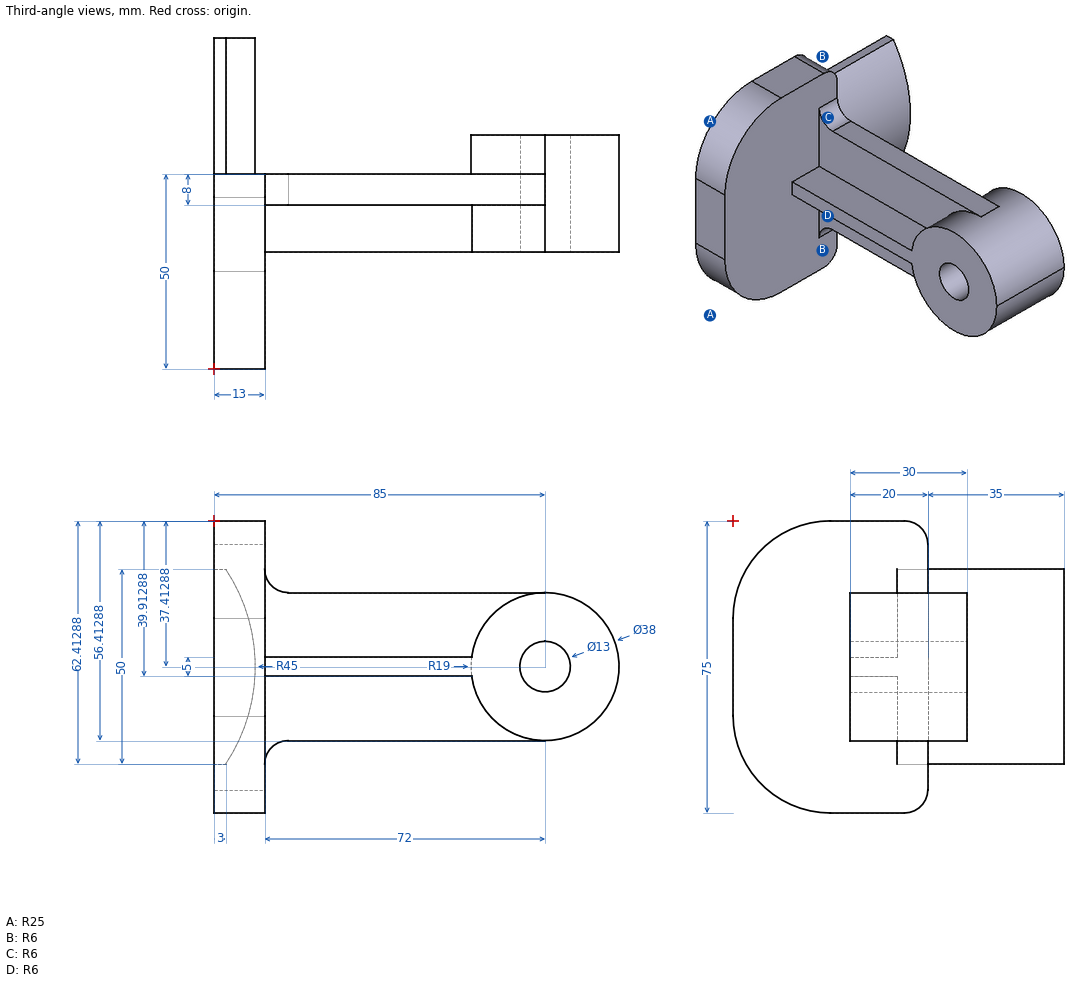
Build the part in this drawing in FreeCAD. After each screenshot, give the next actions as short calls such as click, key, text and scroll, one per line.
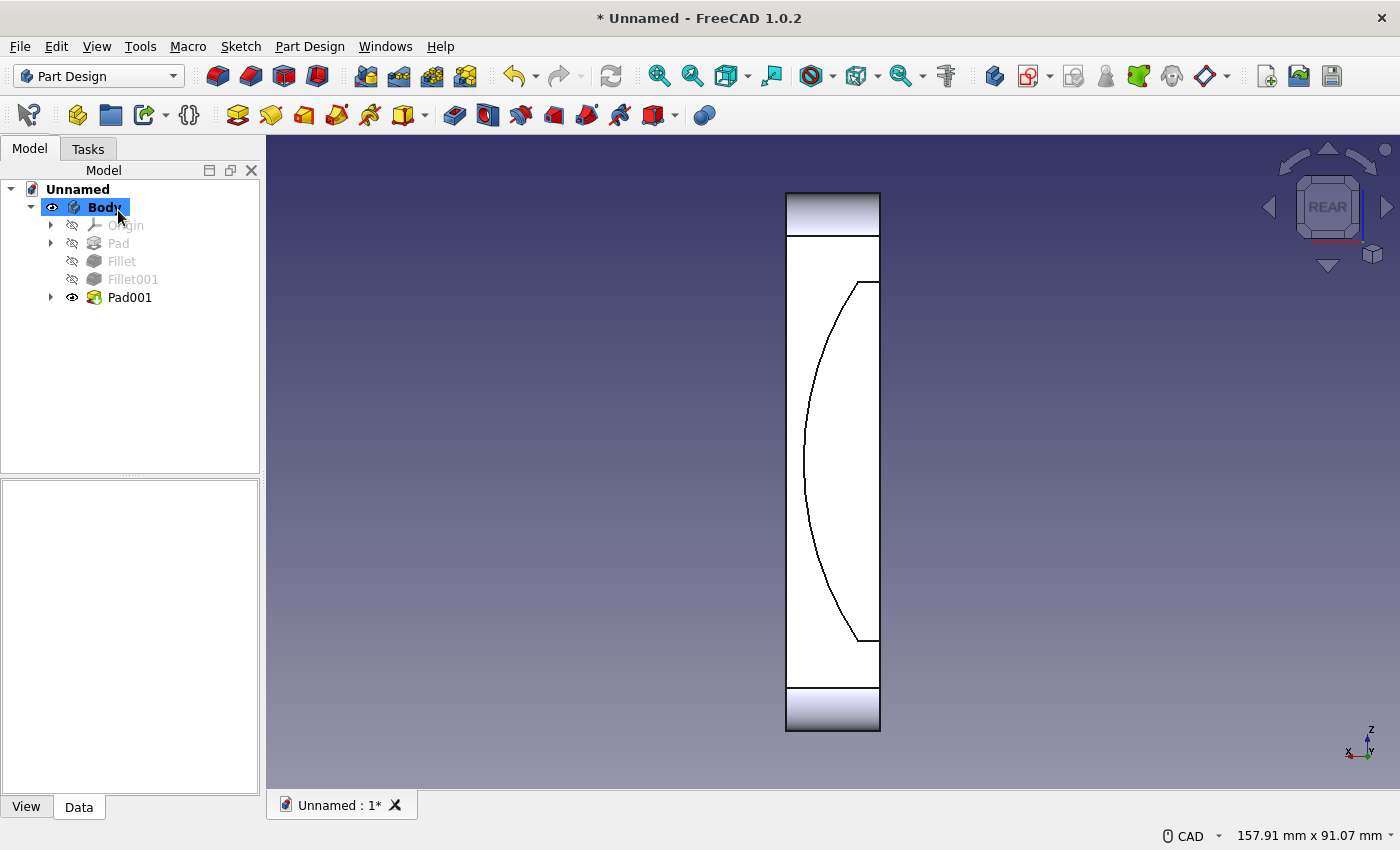
click(995, 76)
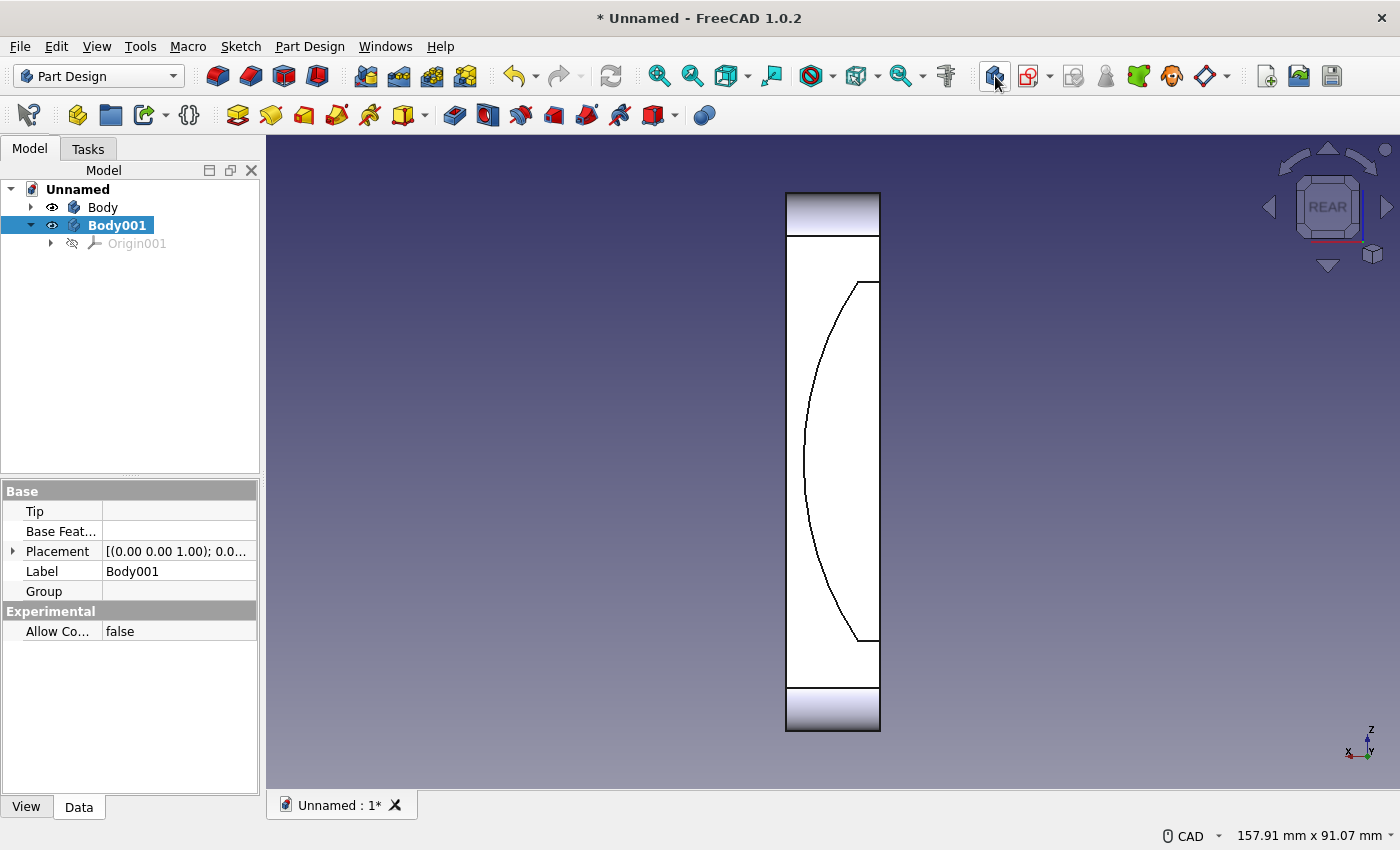
click(51, 243)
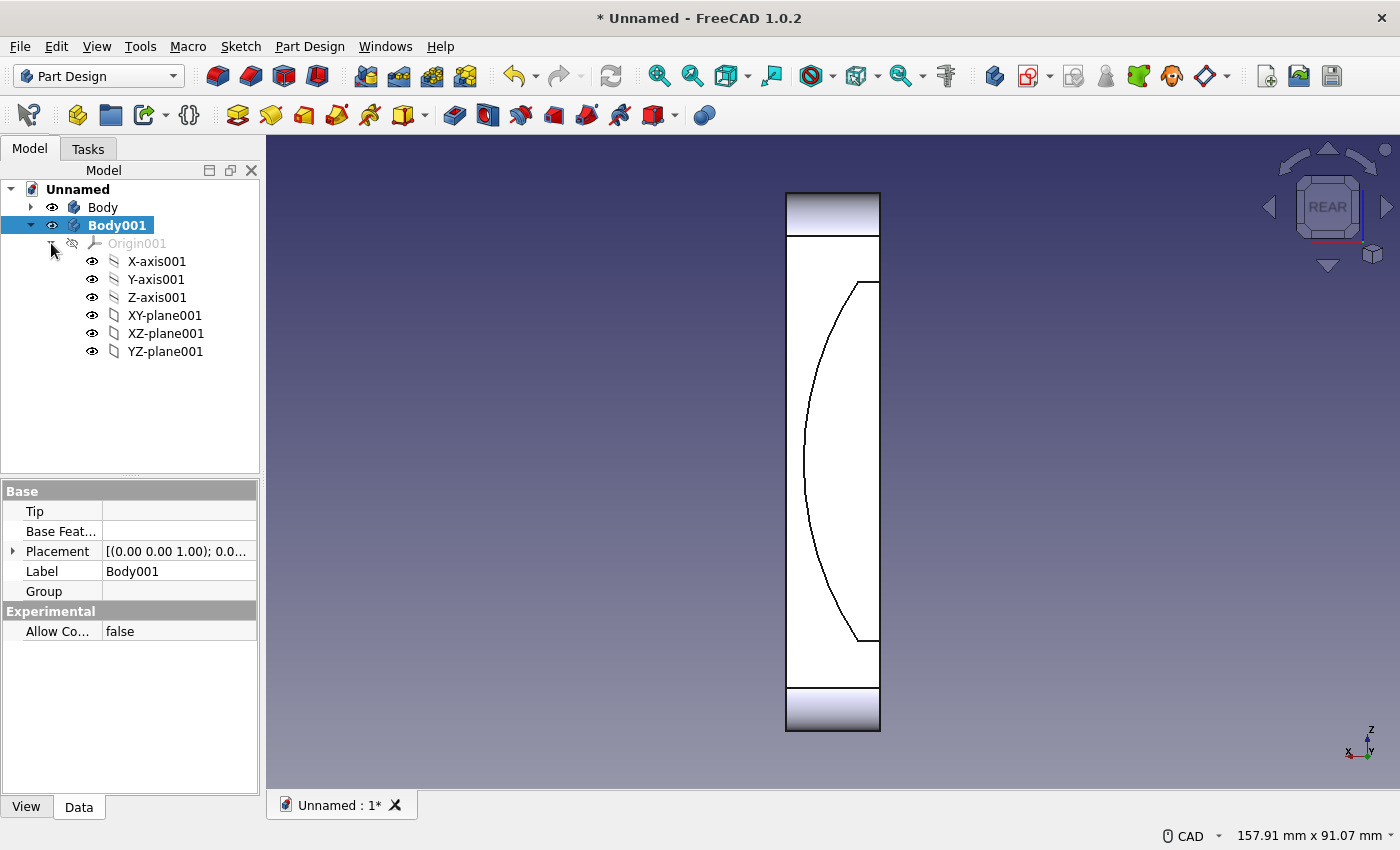
click(137, 333)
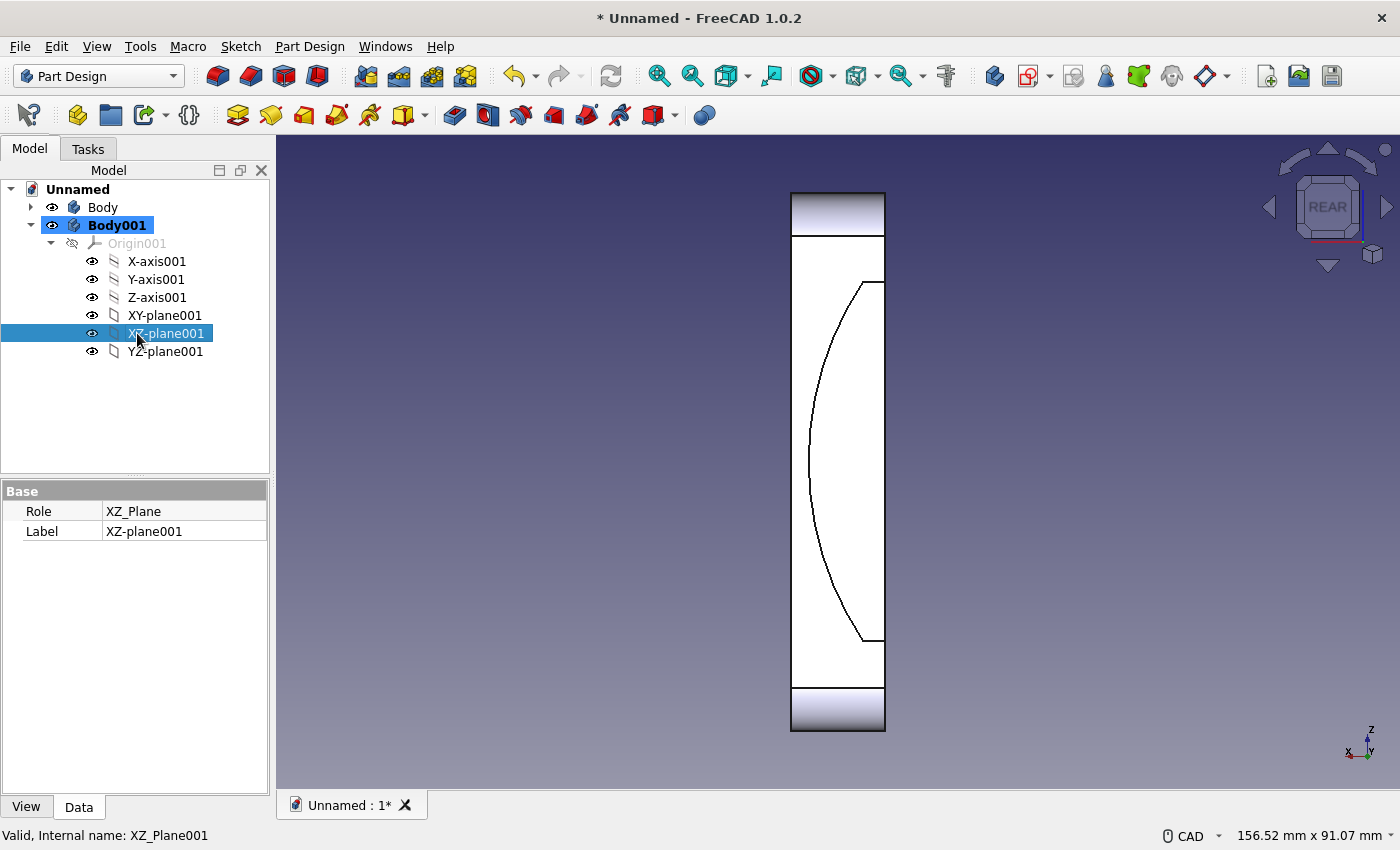
click(1204, 76)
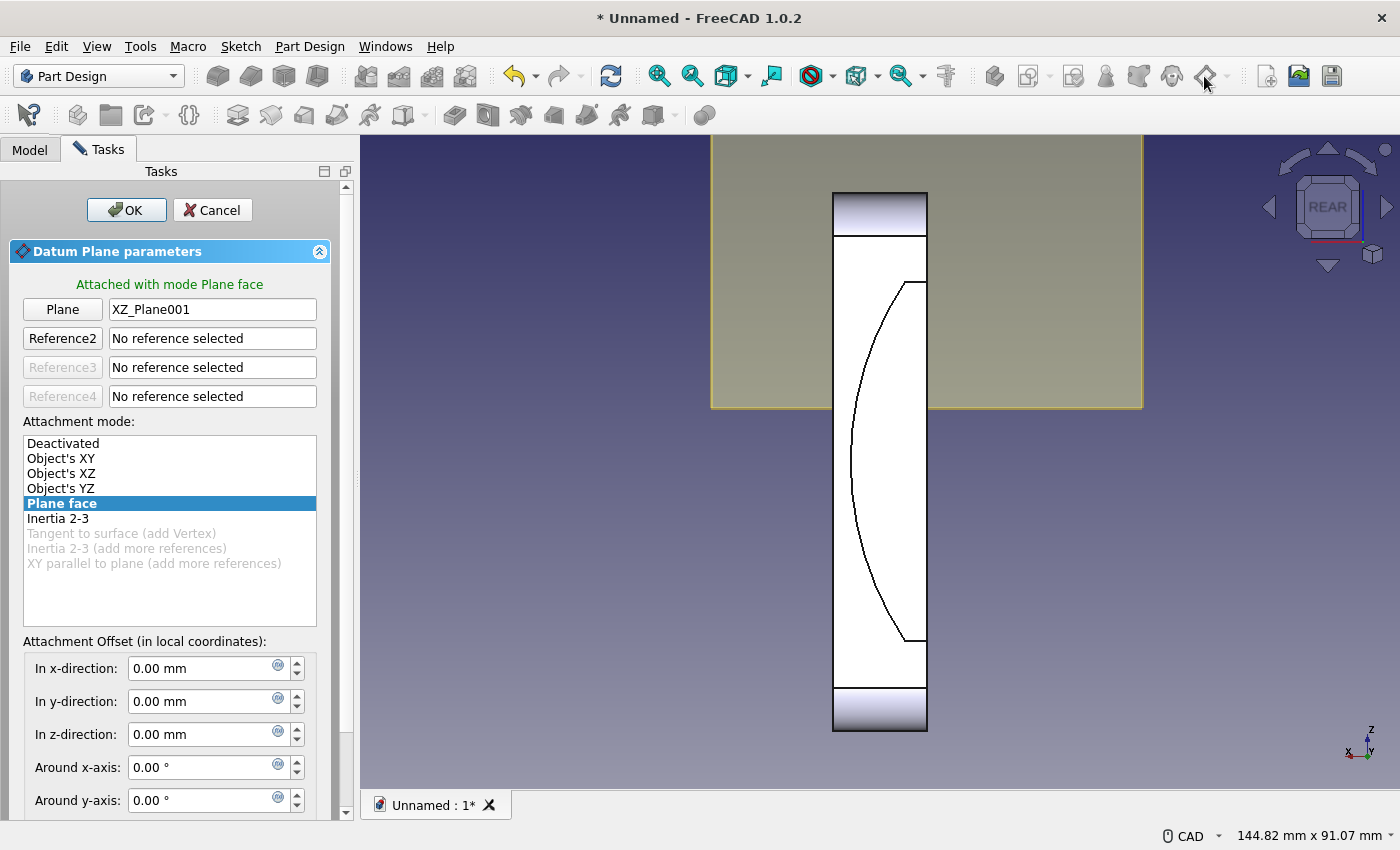
triple_click(210, 734)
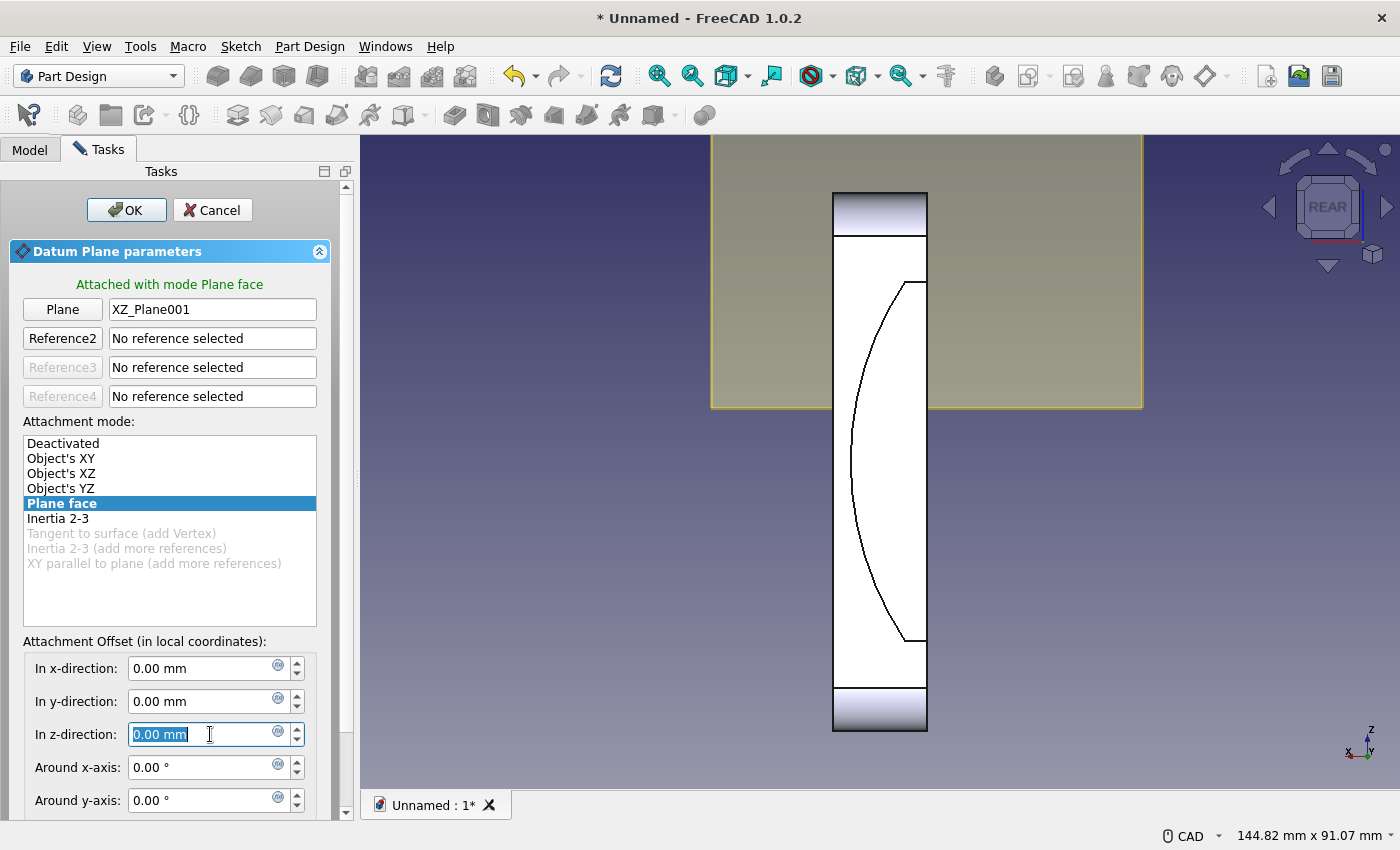
text(-30)
key(Tab)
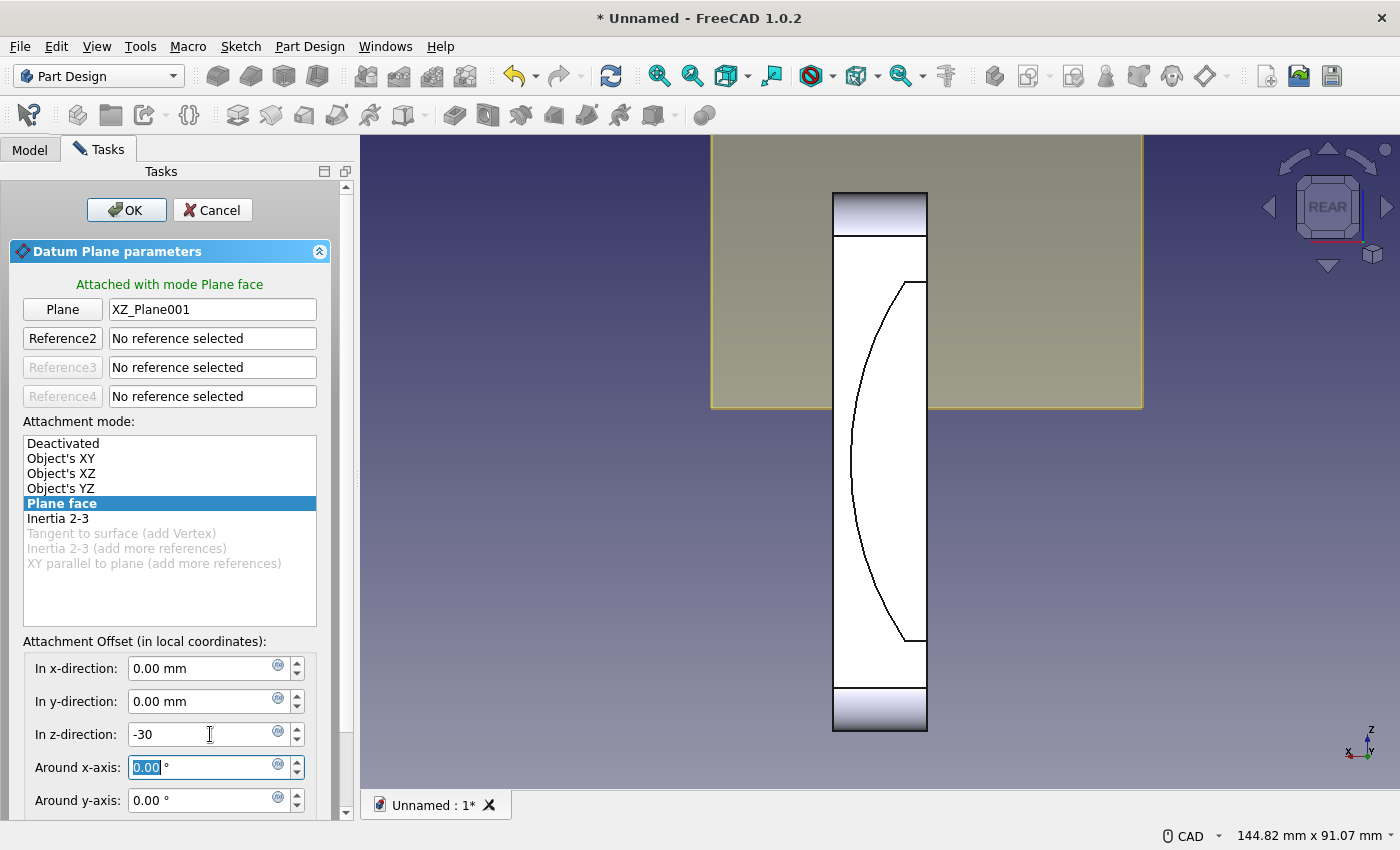
click(127, 210)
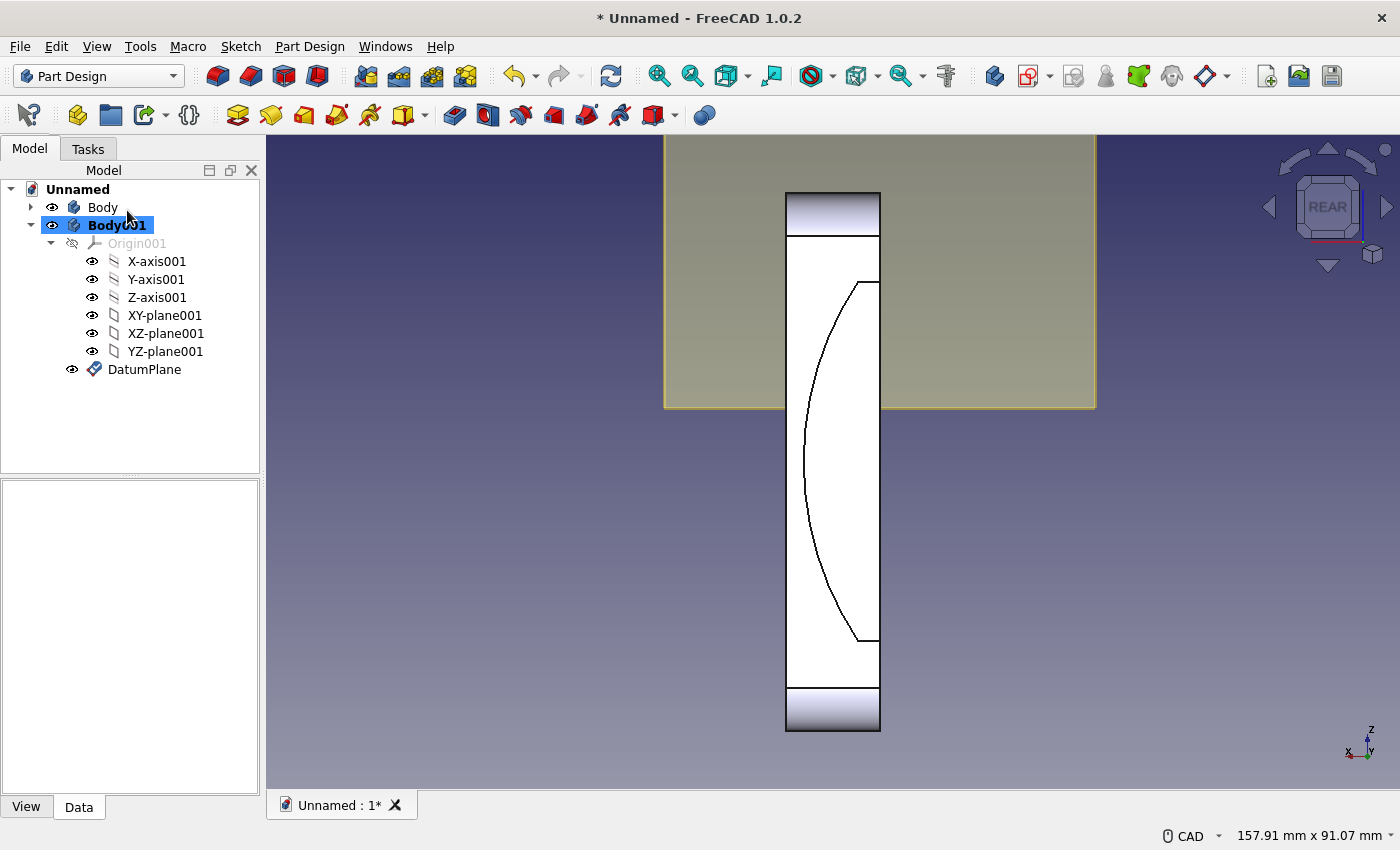
click(117, 369)